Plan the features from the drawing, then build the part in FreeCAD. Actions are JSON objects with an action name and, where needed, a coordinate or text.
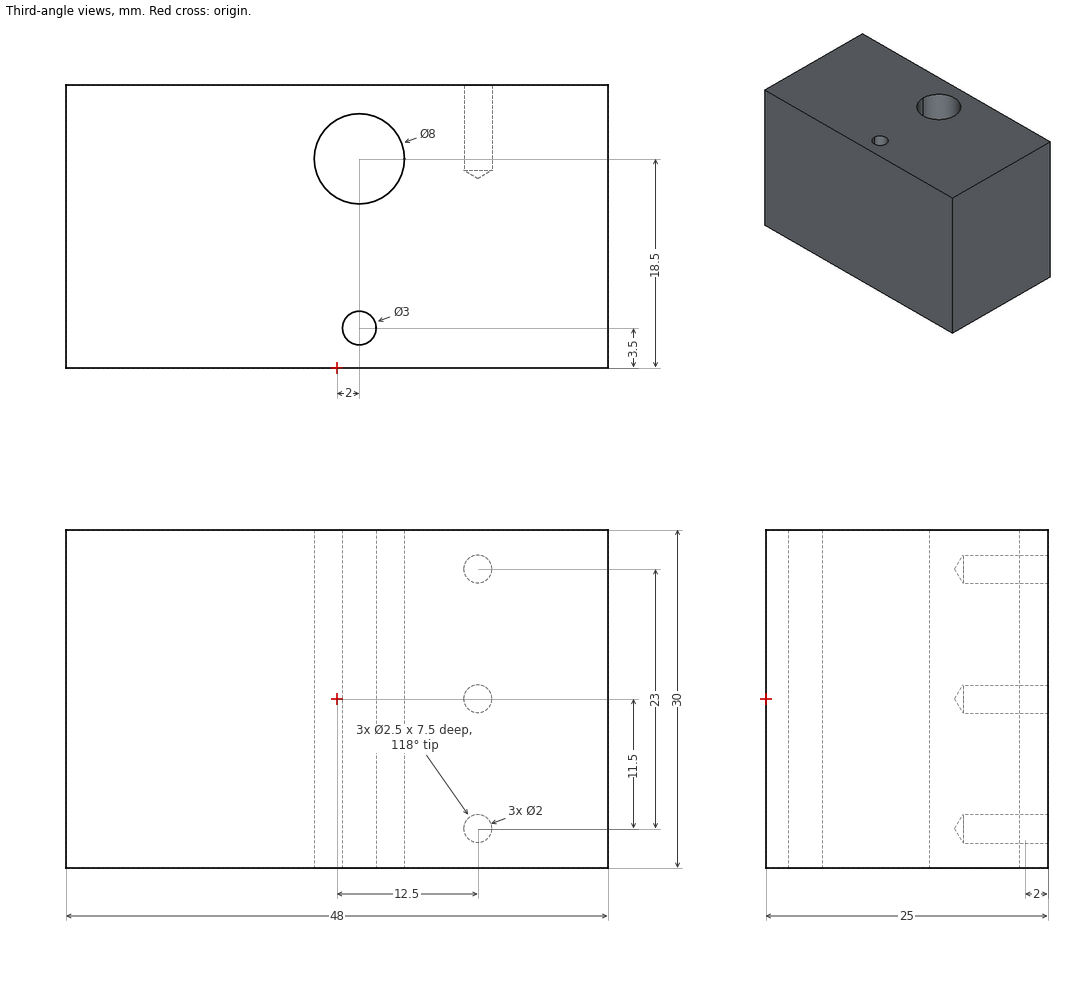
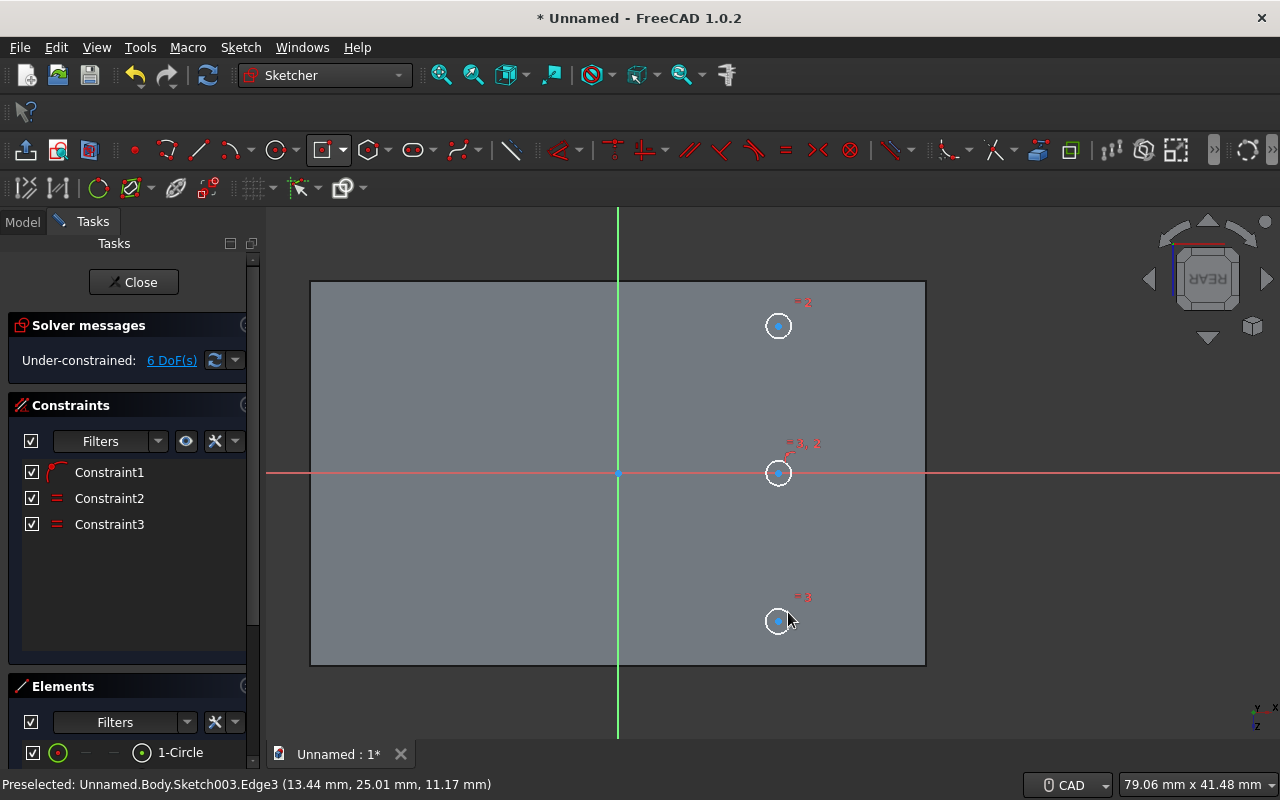
{"action": "left_click", "coordinate": [779, 326]}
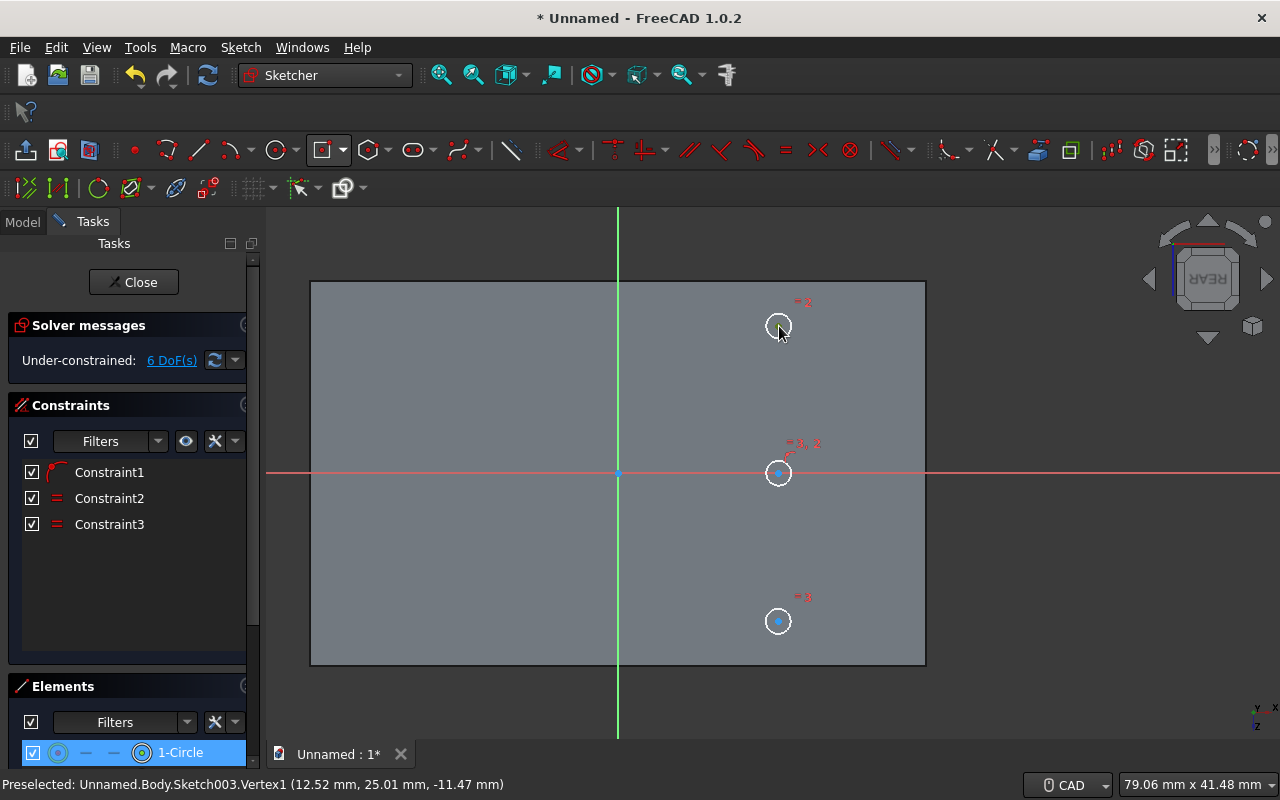
{"action": "left_click", "coordinate": [779, 473]}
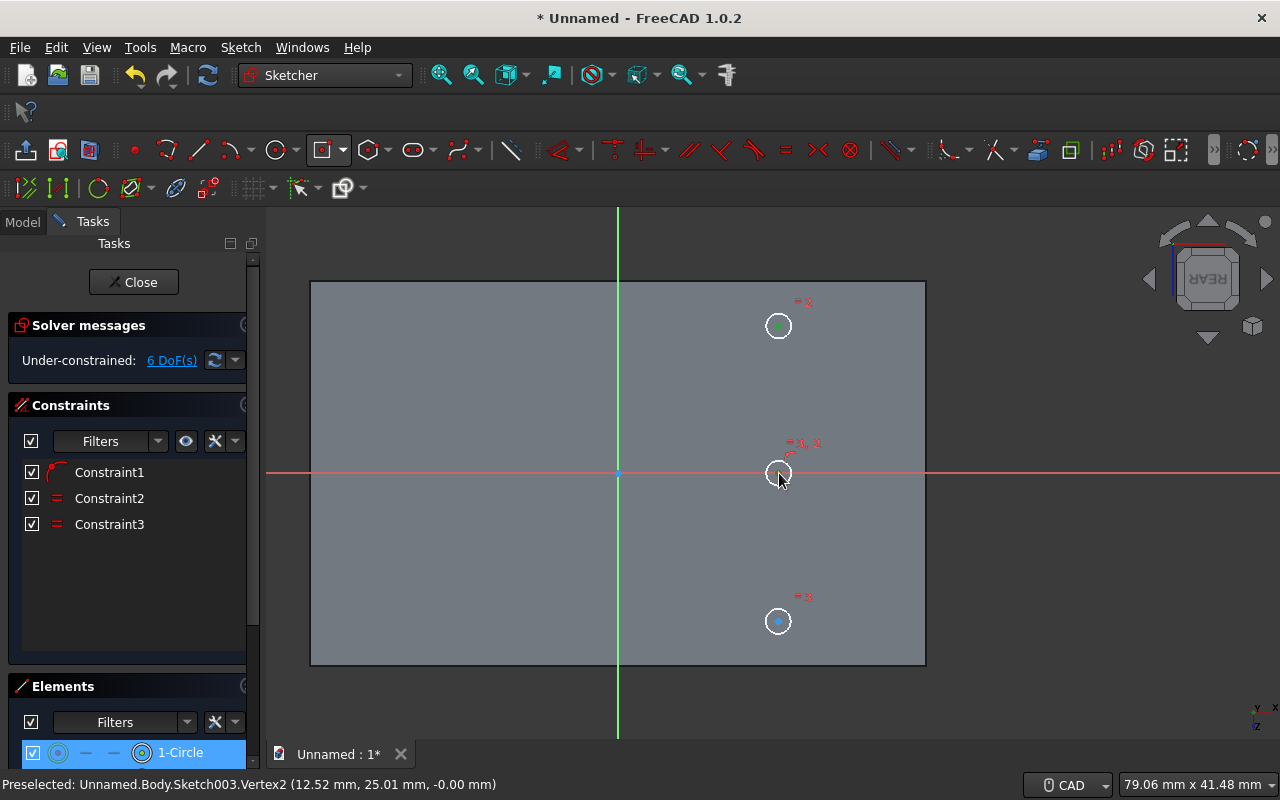
{"action": "key", "text": "v"}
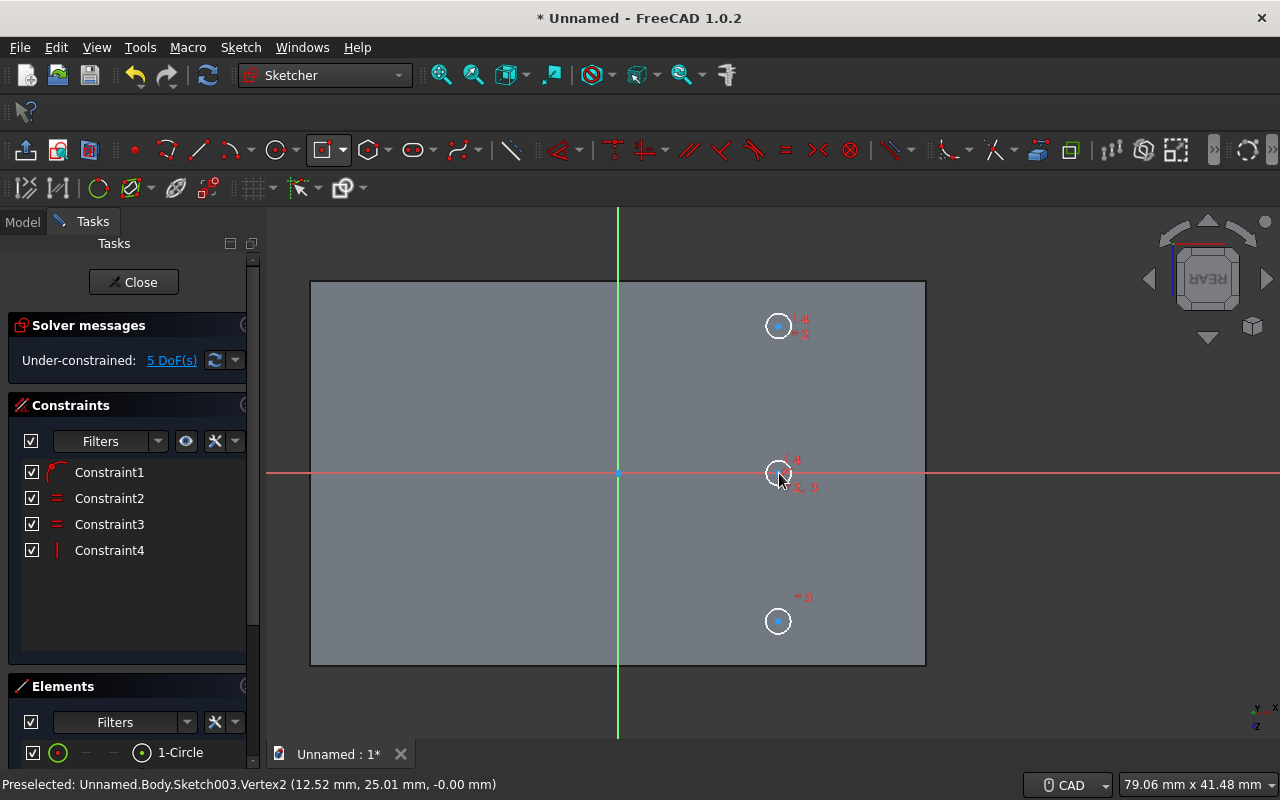
{"action": "left_click", "coordinate": [779, 473]}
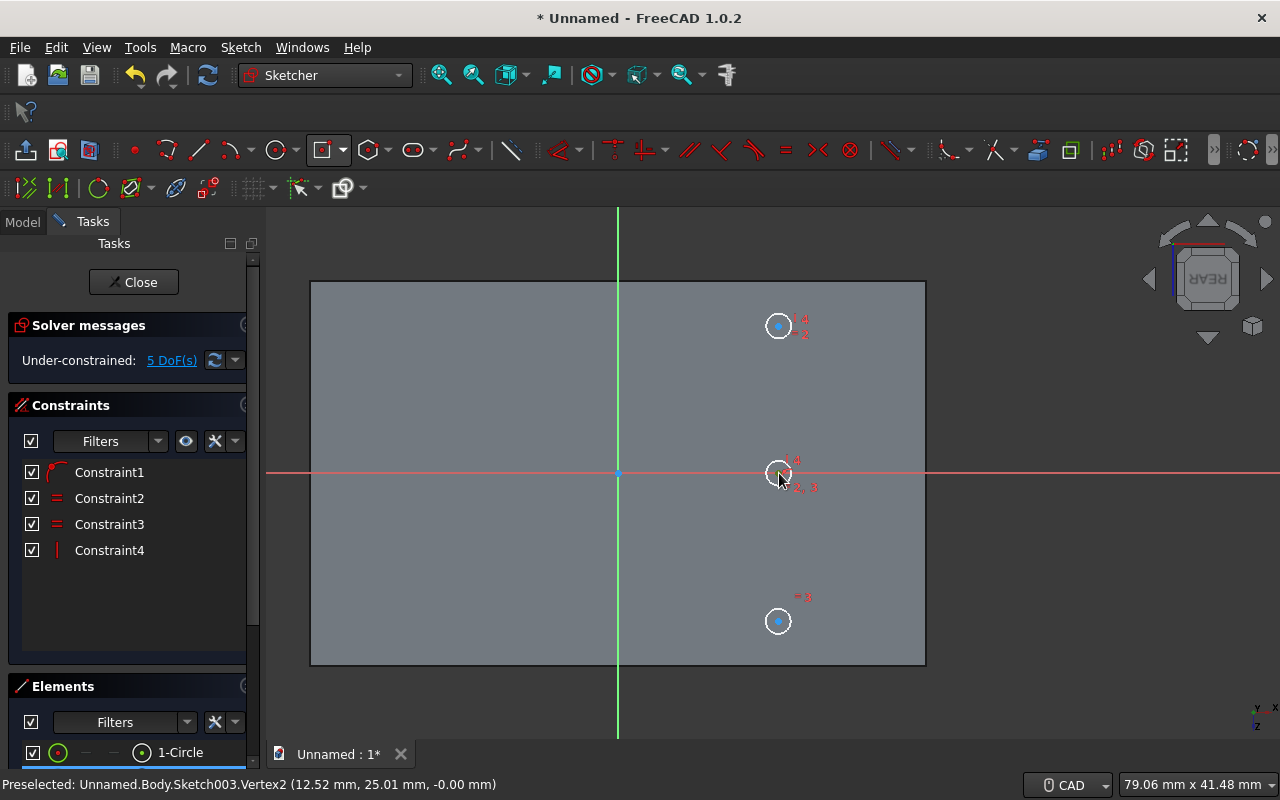
{"action": "left_click", "coordinate": [778, 621]}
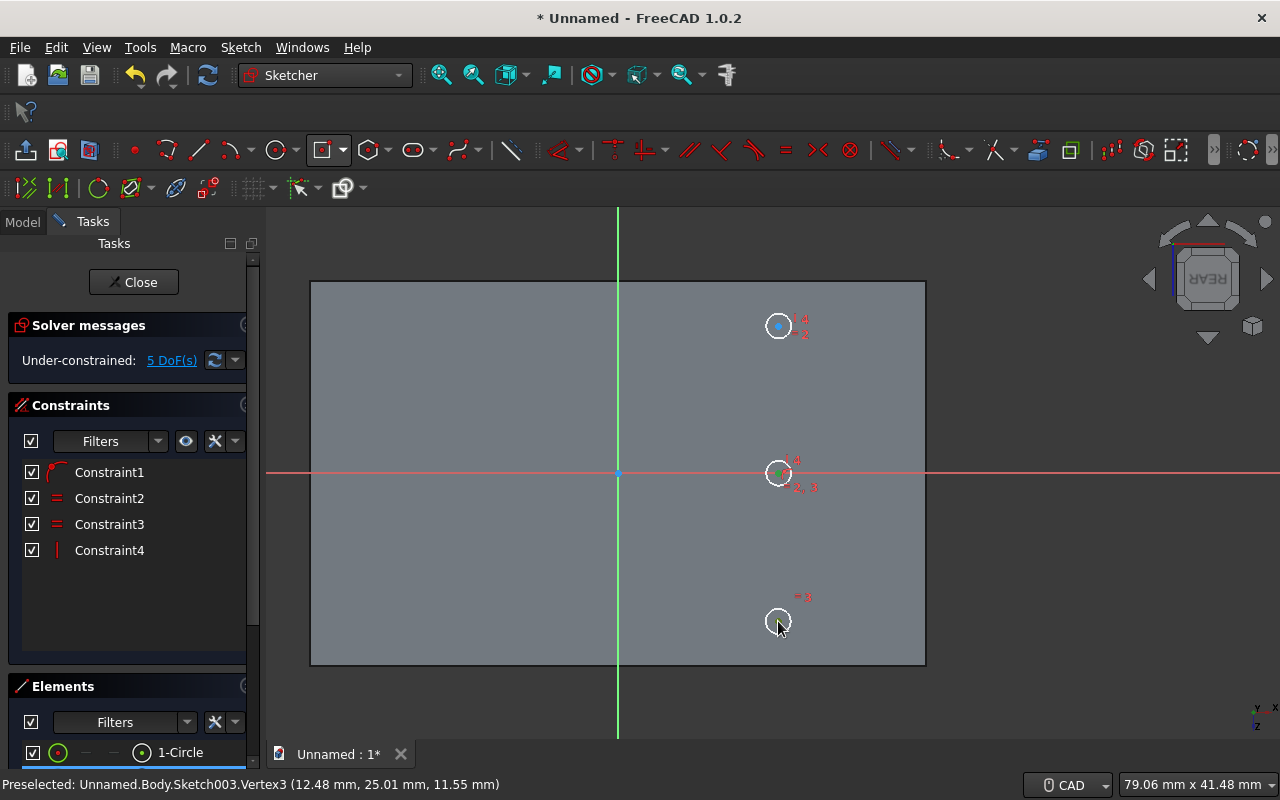
{"action": "key", "text": "v"}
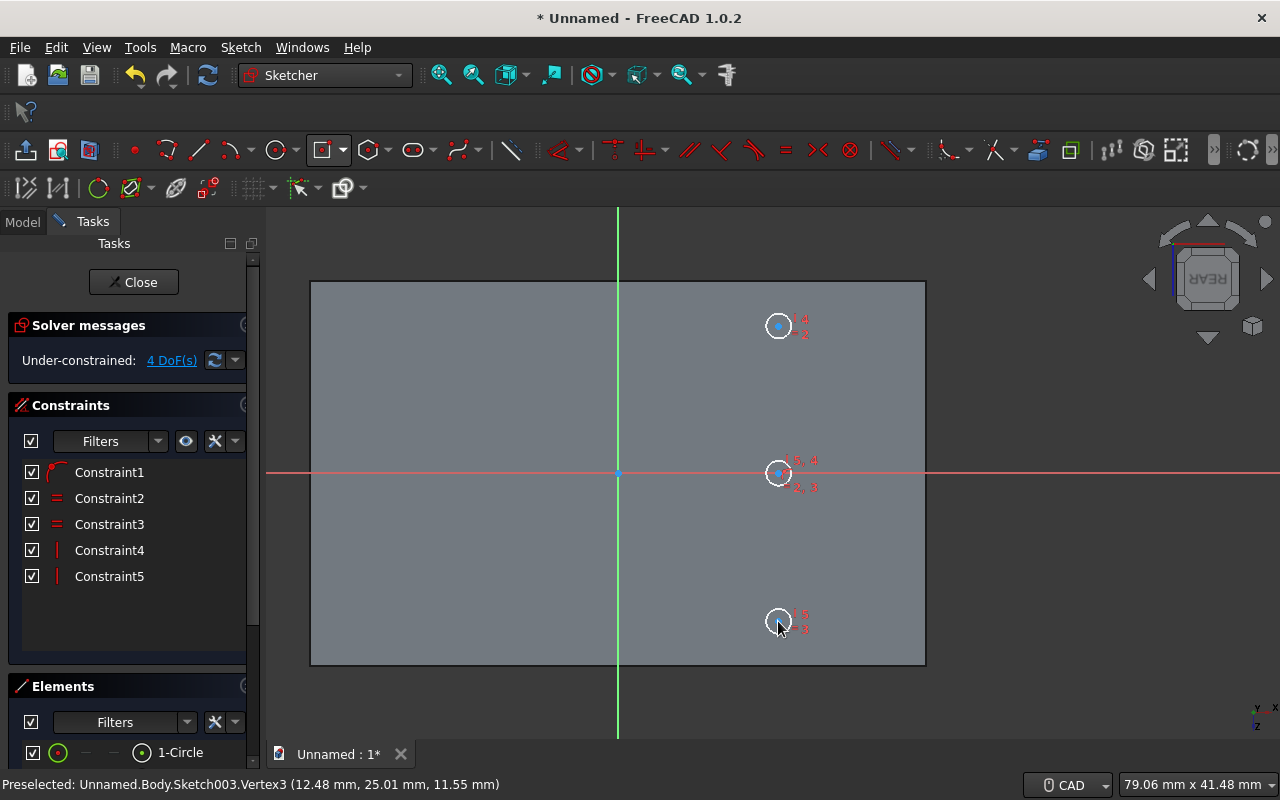
{"action": "left_click", "coordinate": [558, 150]}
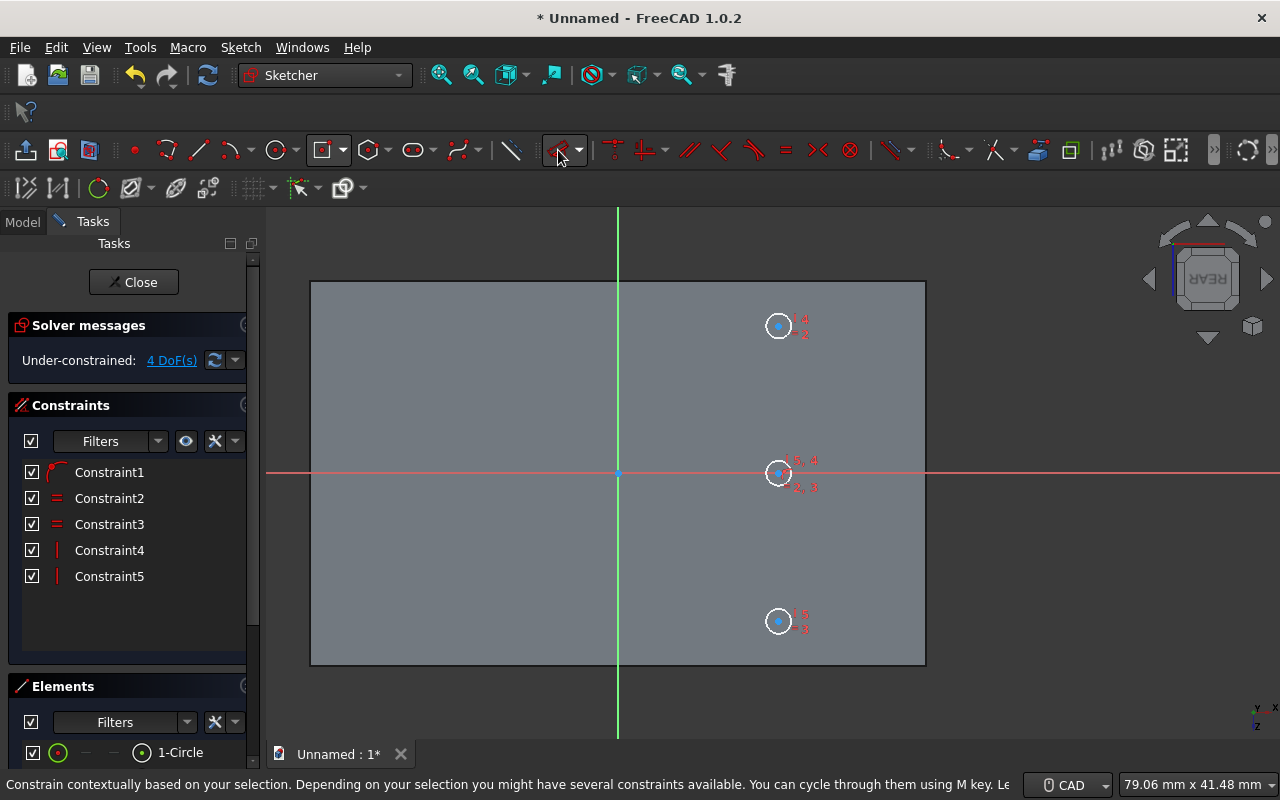
{"action": "scroll", "coordinate": [787, 317], "scroll_direction": "up", "scroll_amount": 3}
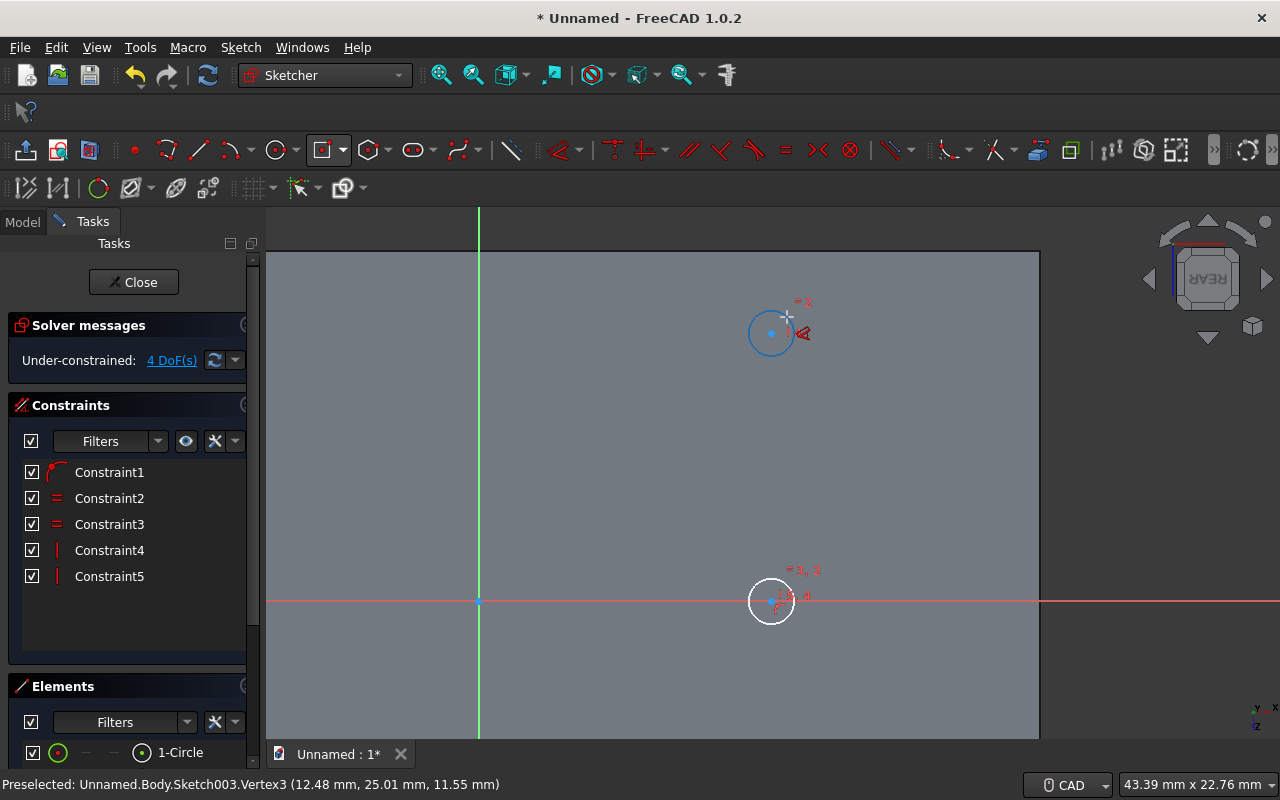
{"action": "left_click", "coordinate": [787, 317]}
{"action": "left_click", "coordinate": [809, 294]}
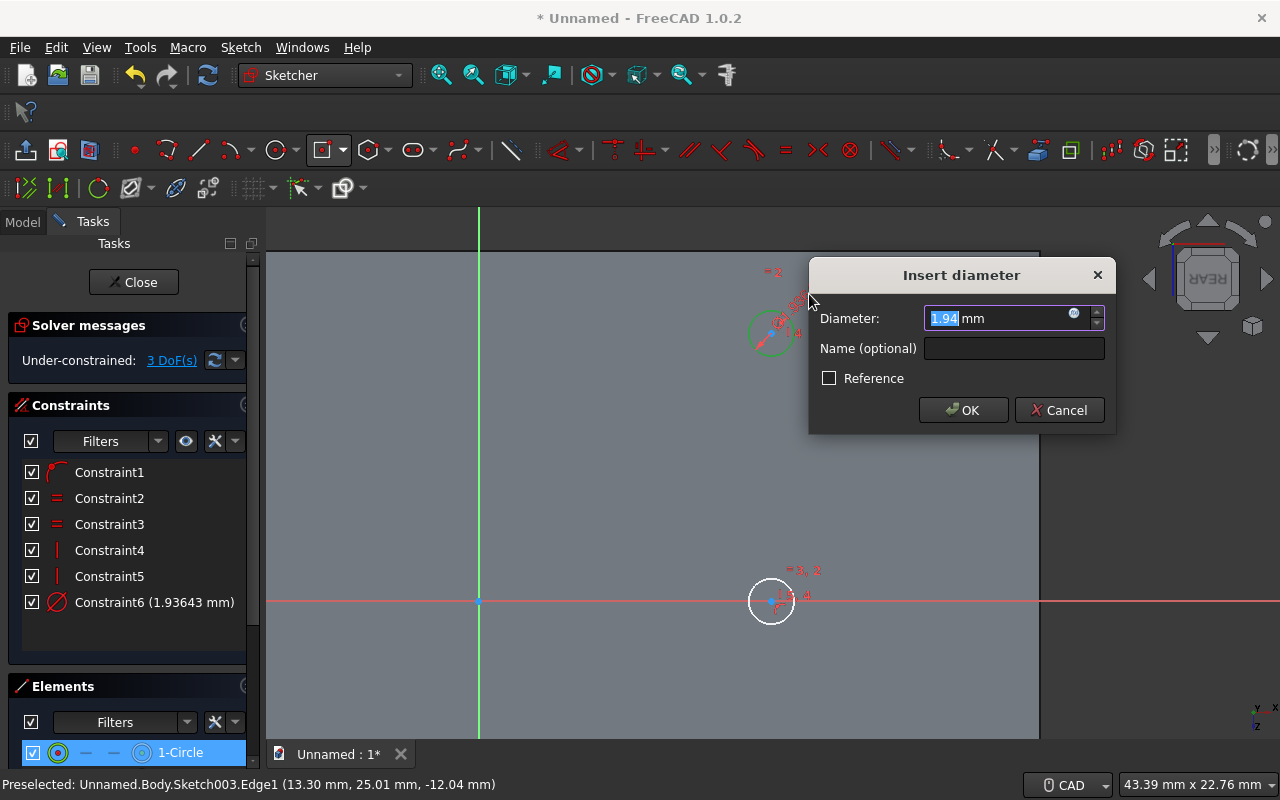
{"action": "type", "text": "2"}
{"action": "key", "text": "Return"}